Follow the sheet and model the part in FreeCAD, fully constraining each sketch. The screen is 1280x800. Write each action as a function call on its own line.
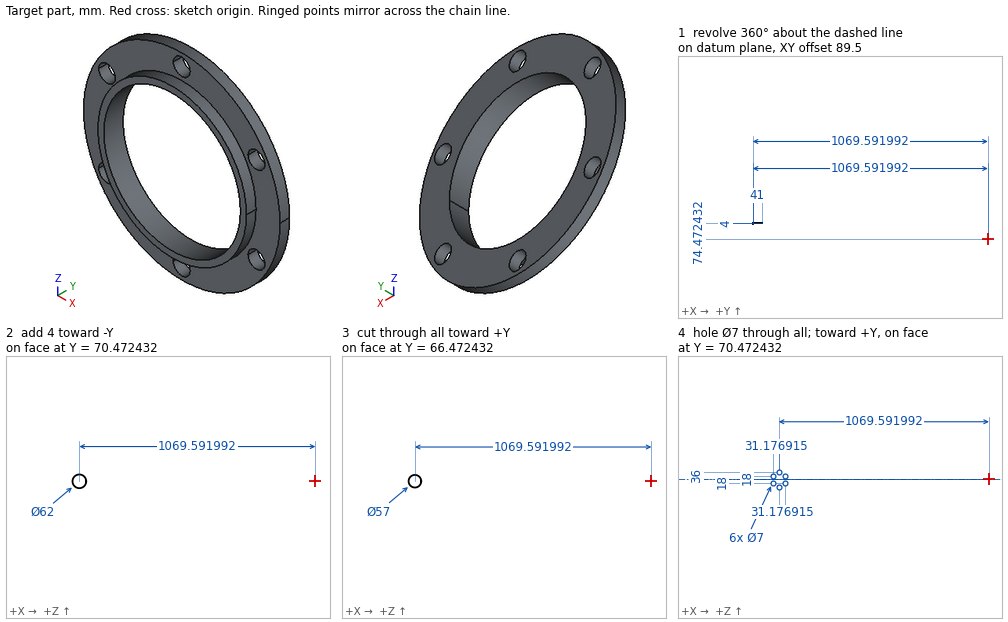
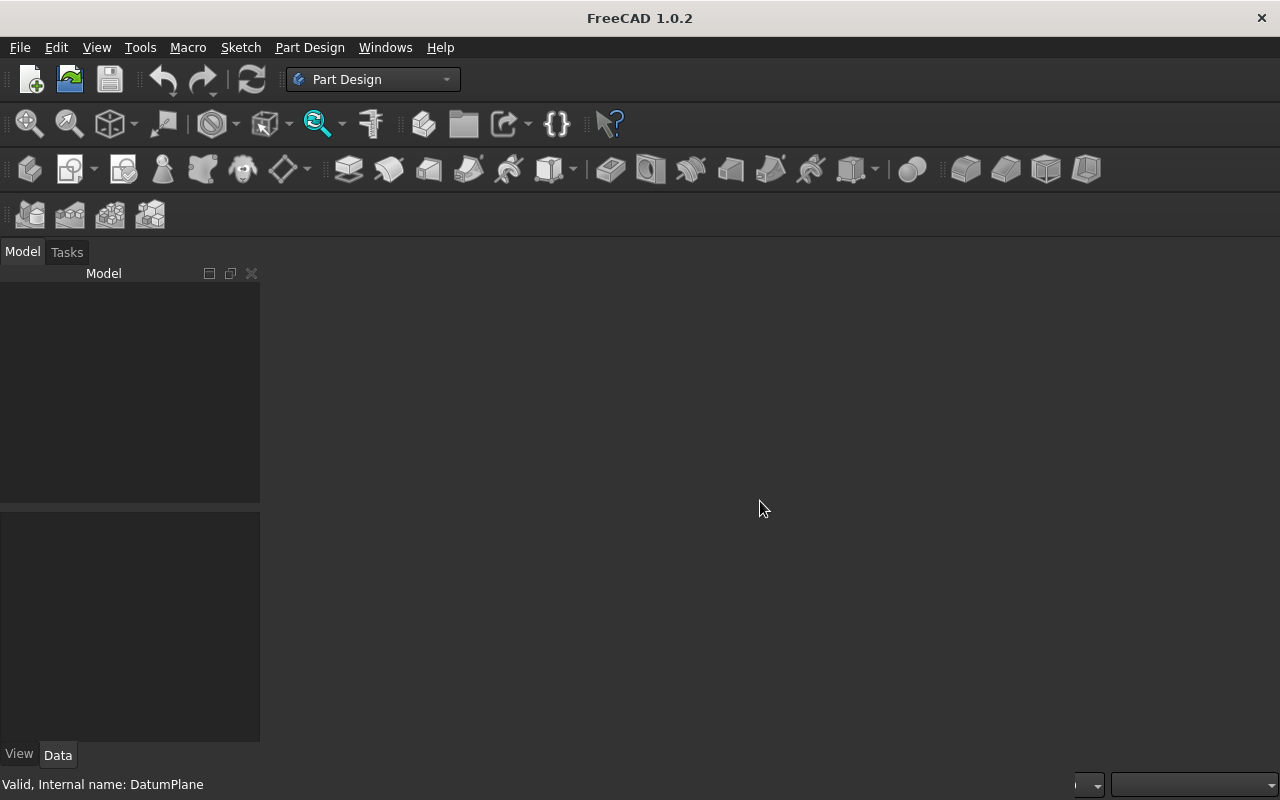
click(30, 80)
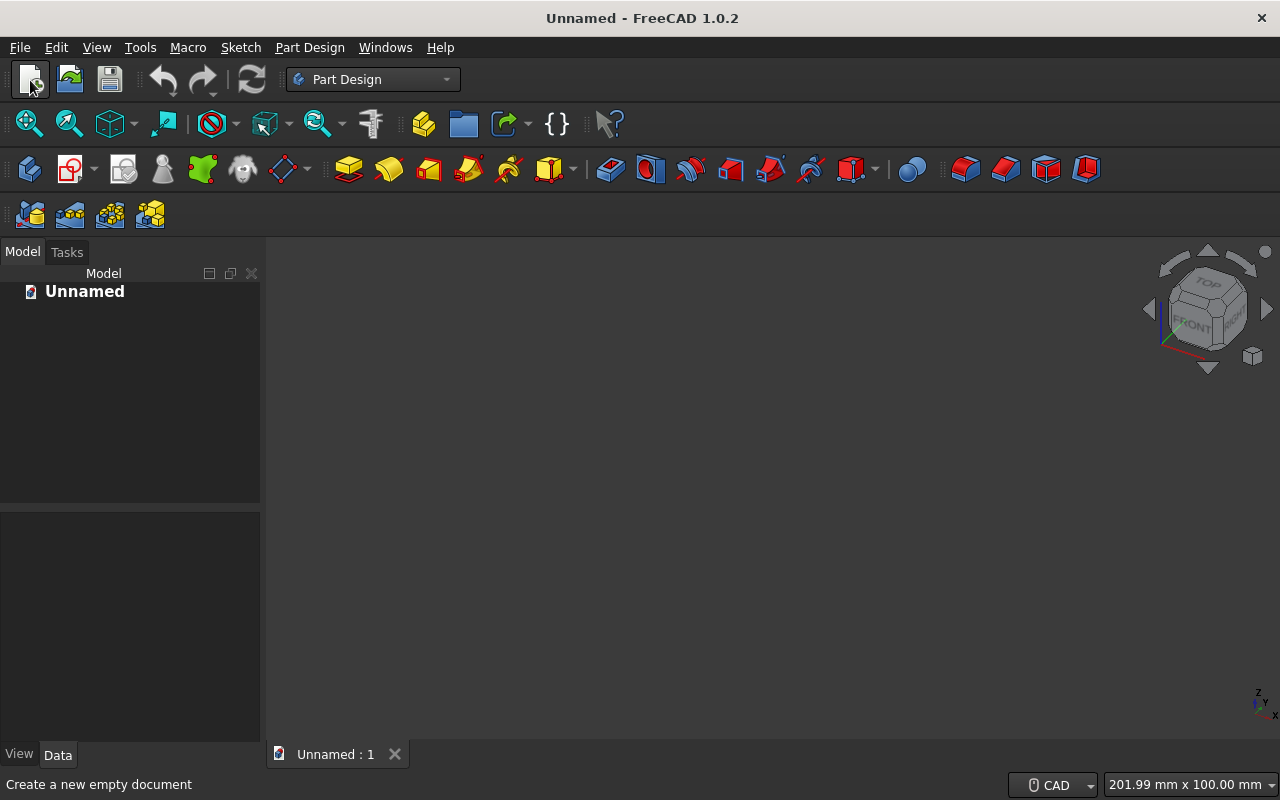
click(30, 170)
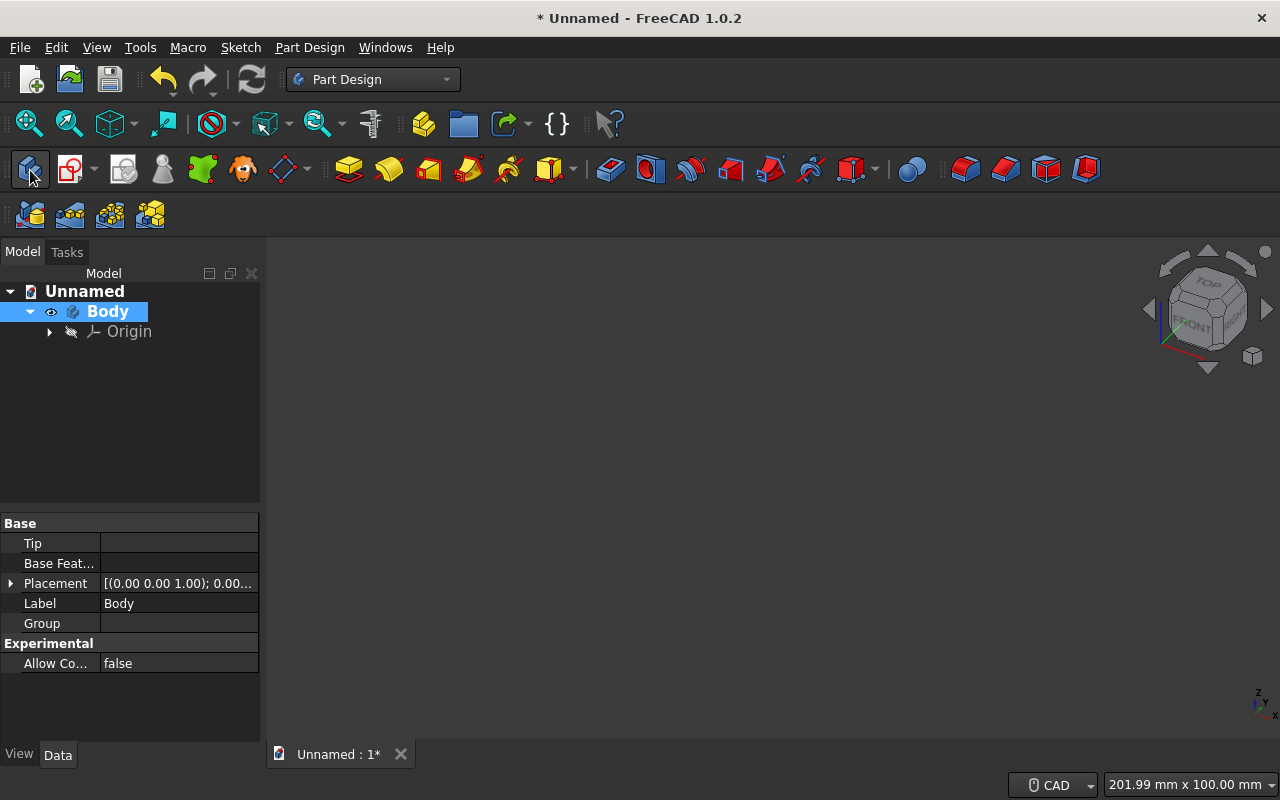
click(50, 332)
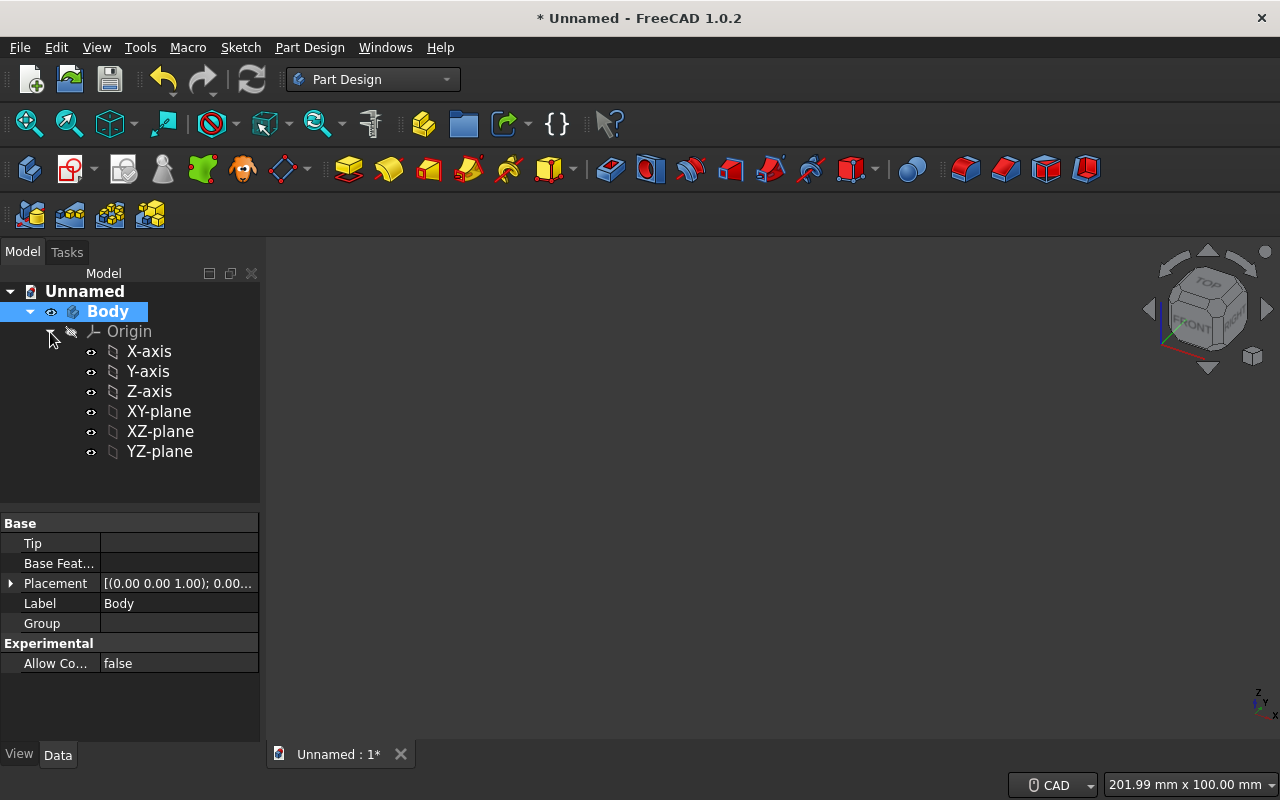
click(136, 412)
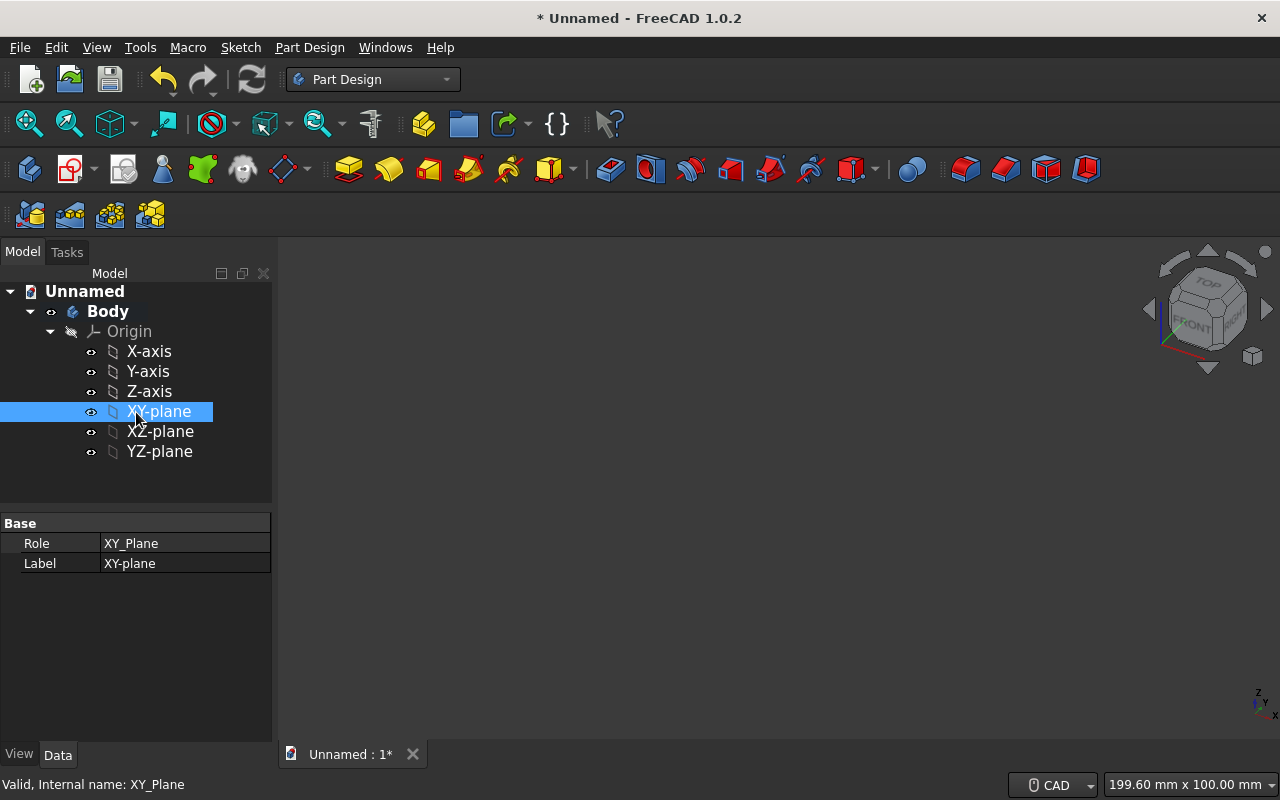
click(284, 170)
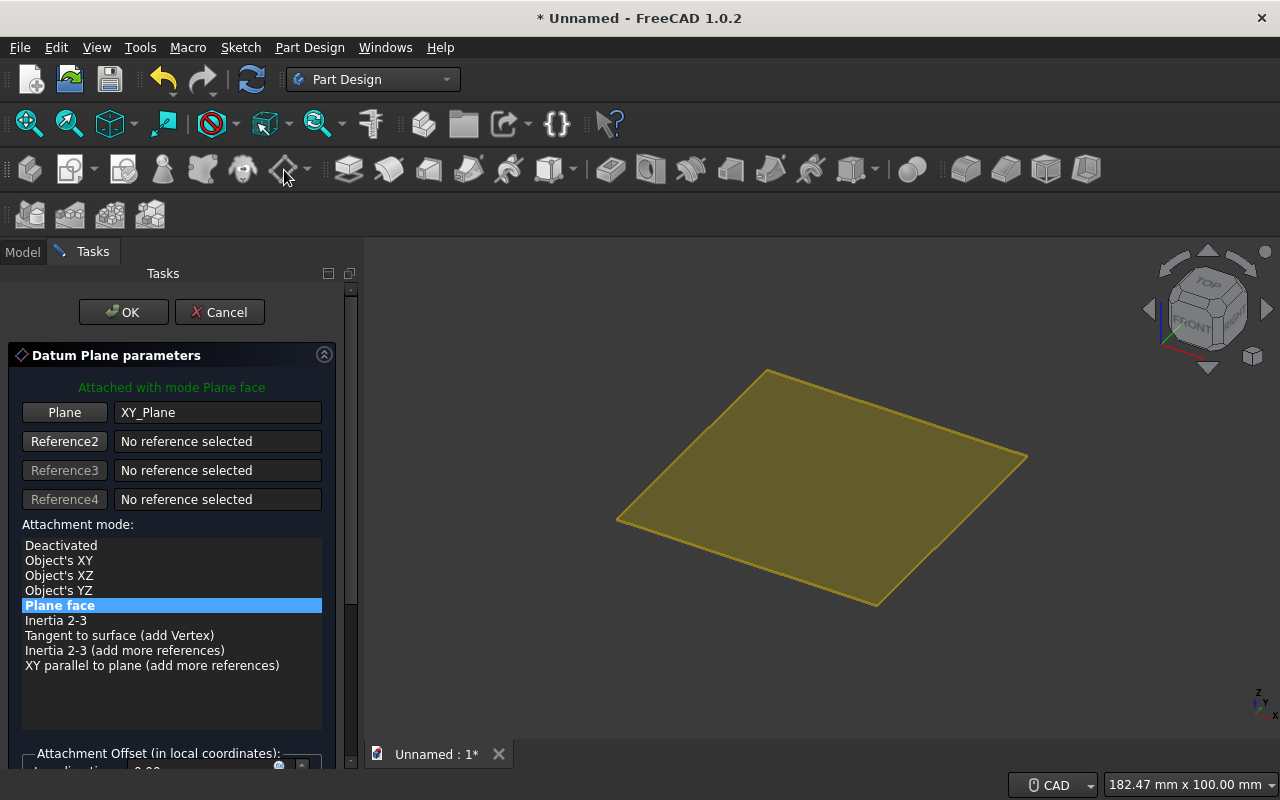
scroll(351, 526, down, 3)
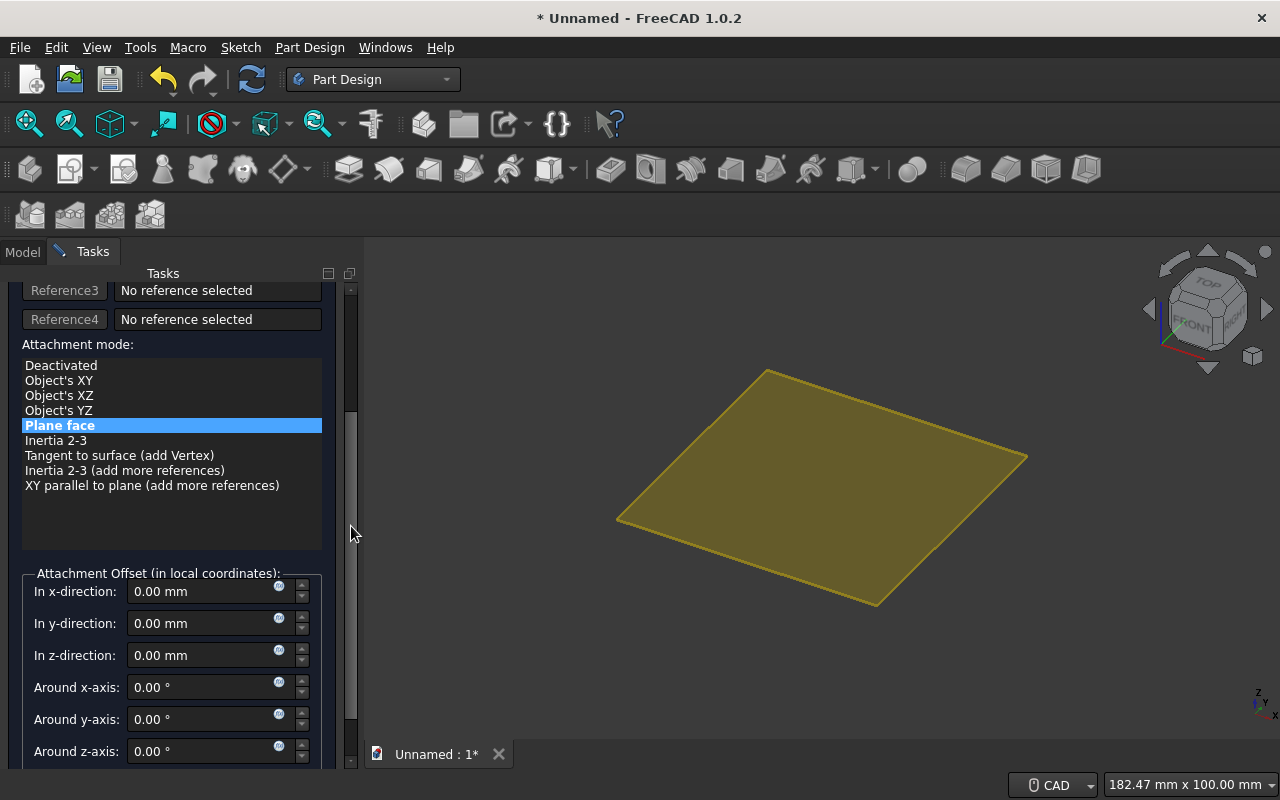
triple_click(210, 655)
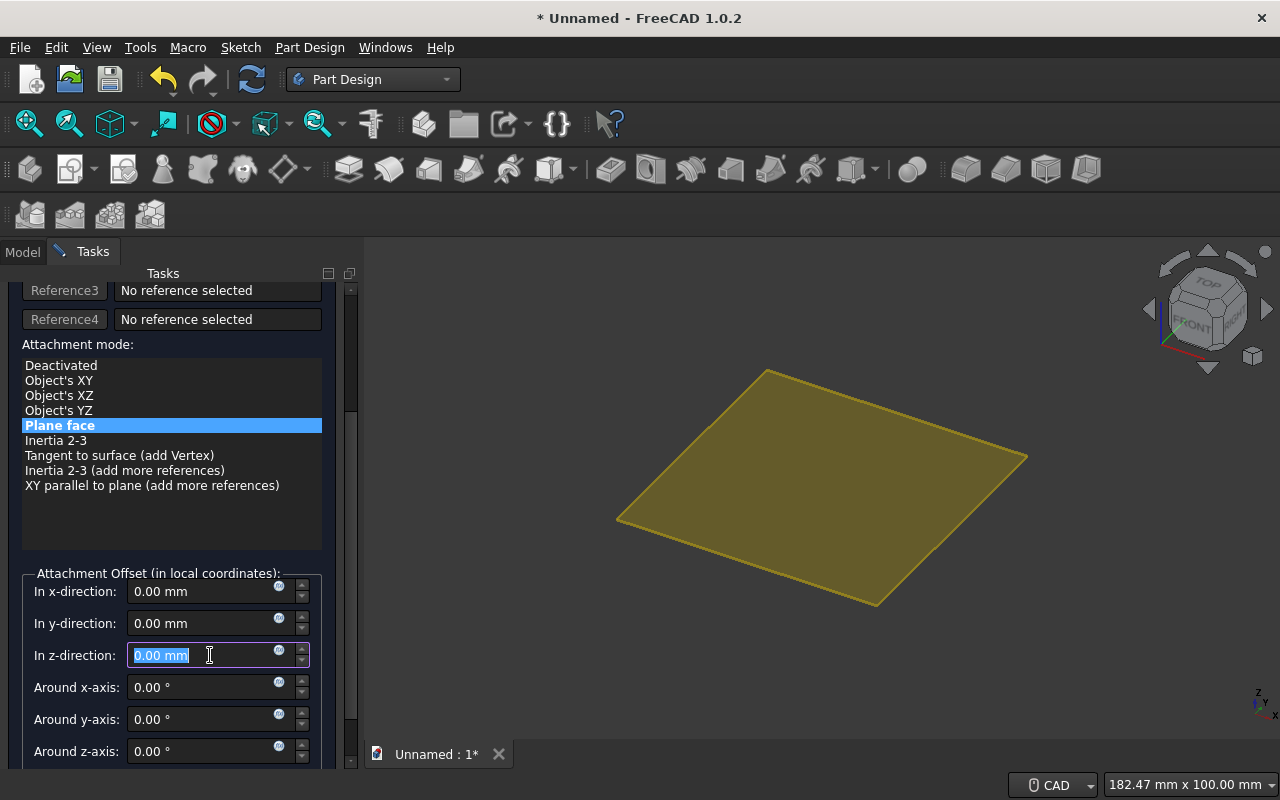
text(89.5)
key(Tab)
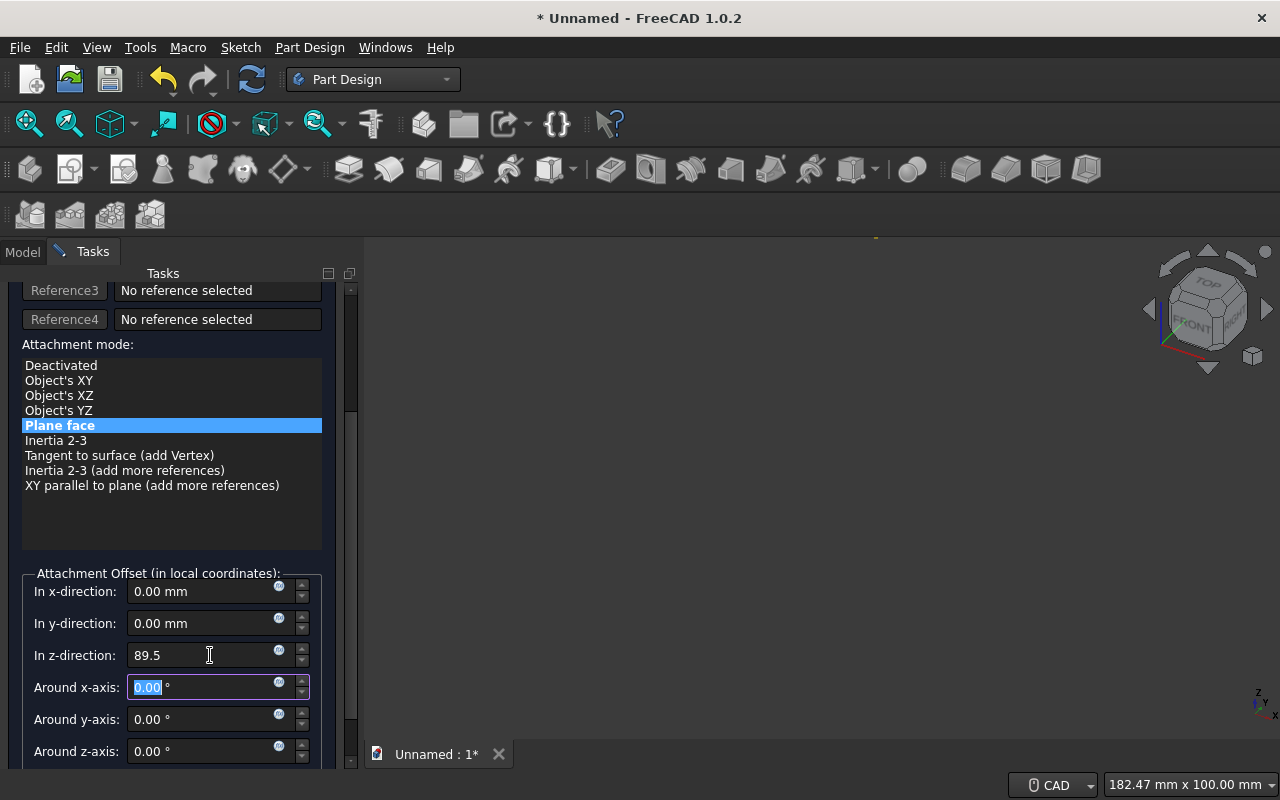
scroll(351, 526, up, 4)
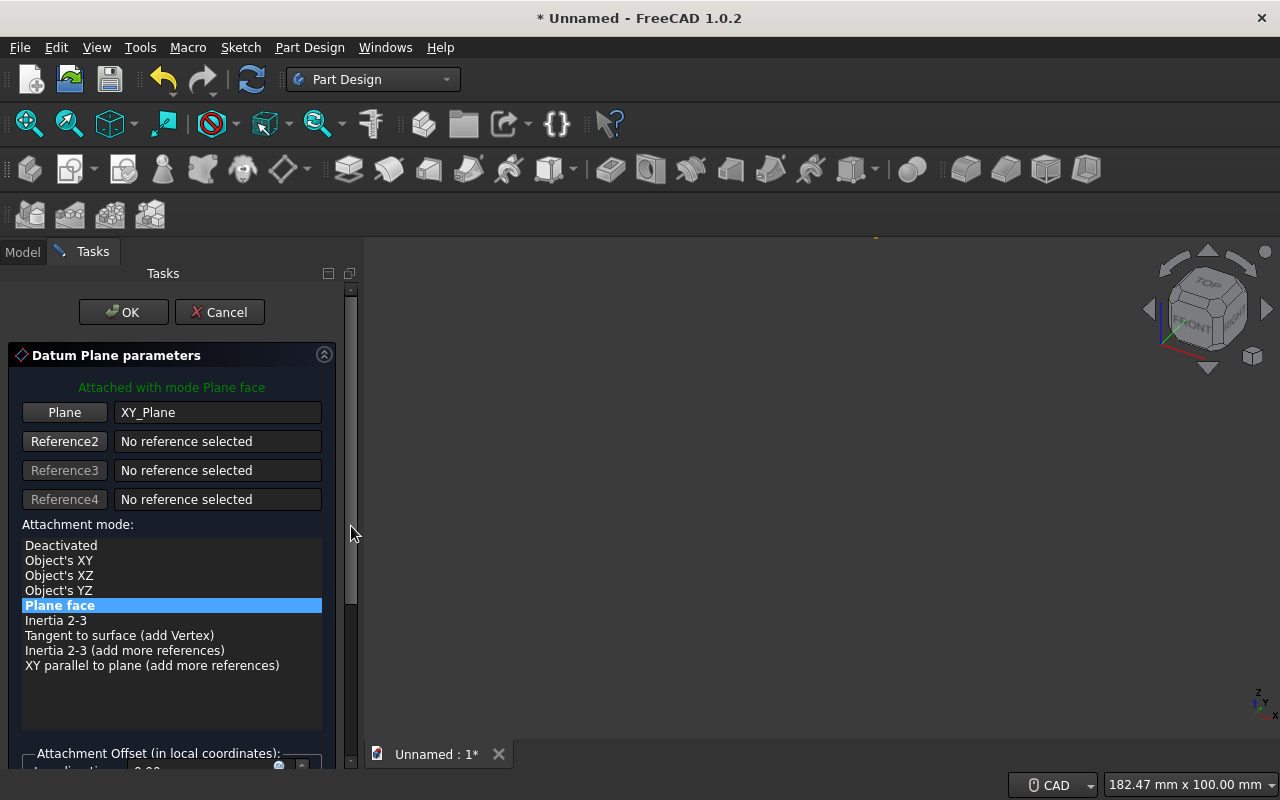
click(124, 312)